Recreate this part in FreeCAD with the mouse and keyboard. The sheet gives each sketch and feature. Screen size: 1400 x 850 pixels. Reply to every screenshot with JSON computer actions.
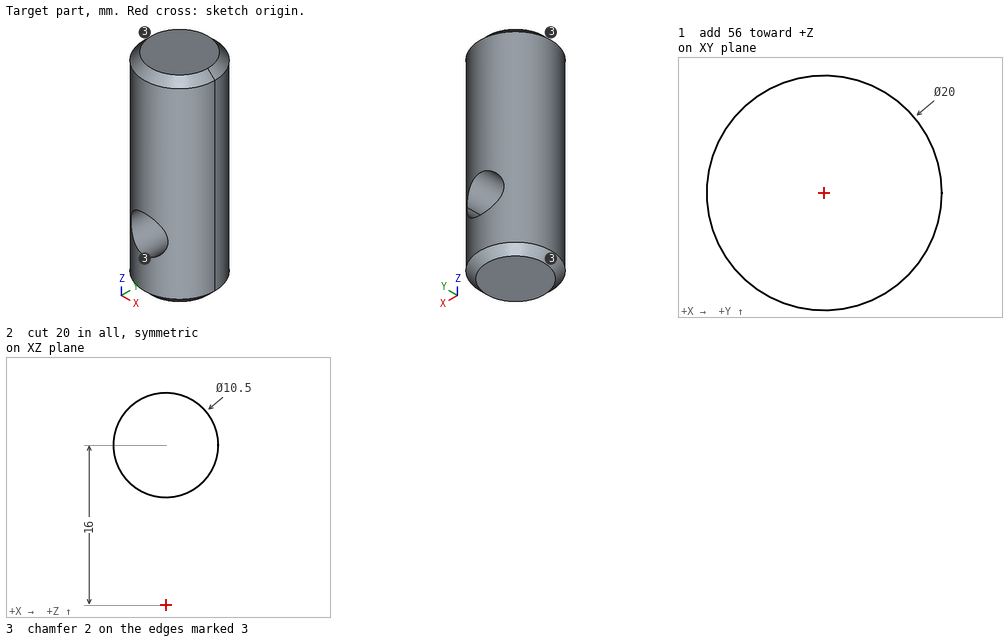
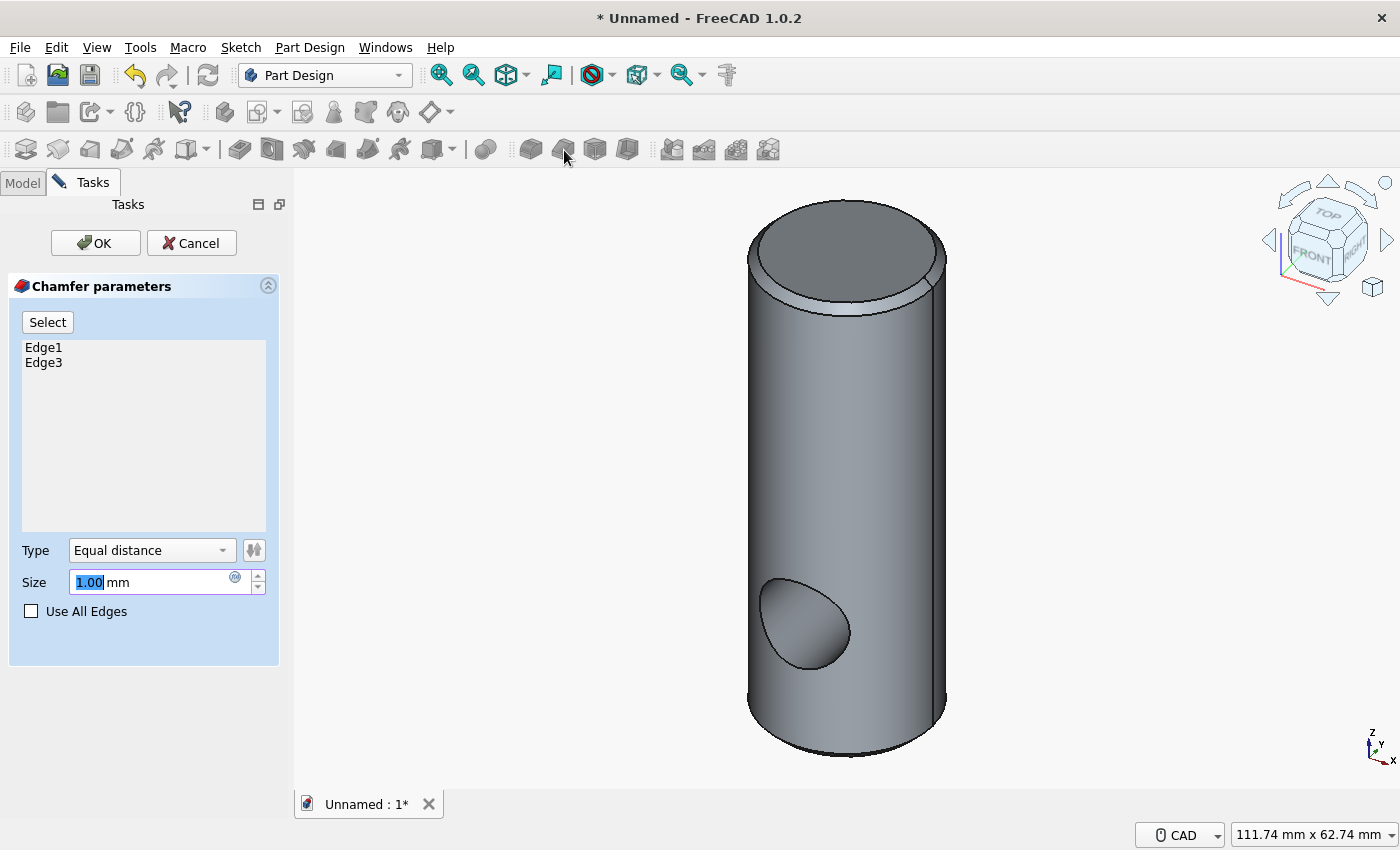
{"action": "type", "text": "2"}
{"action": "key", "text": "Tab"}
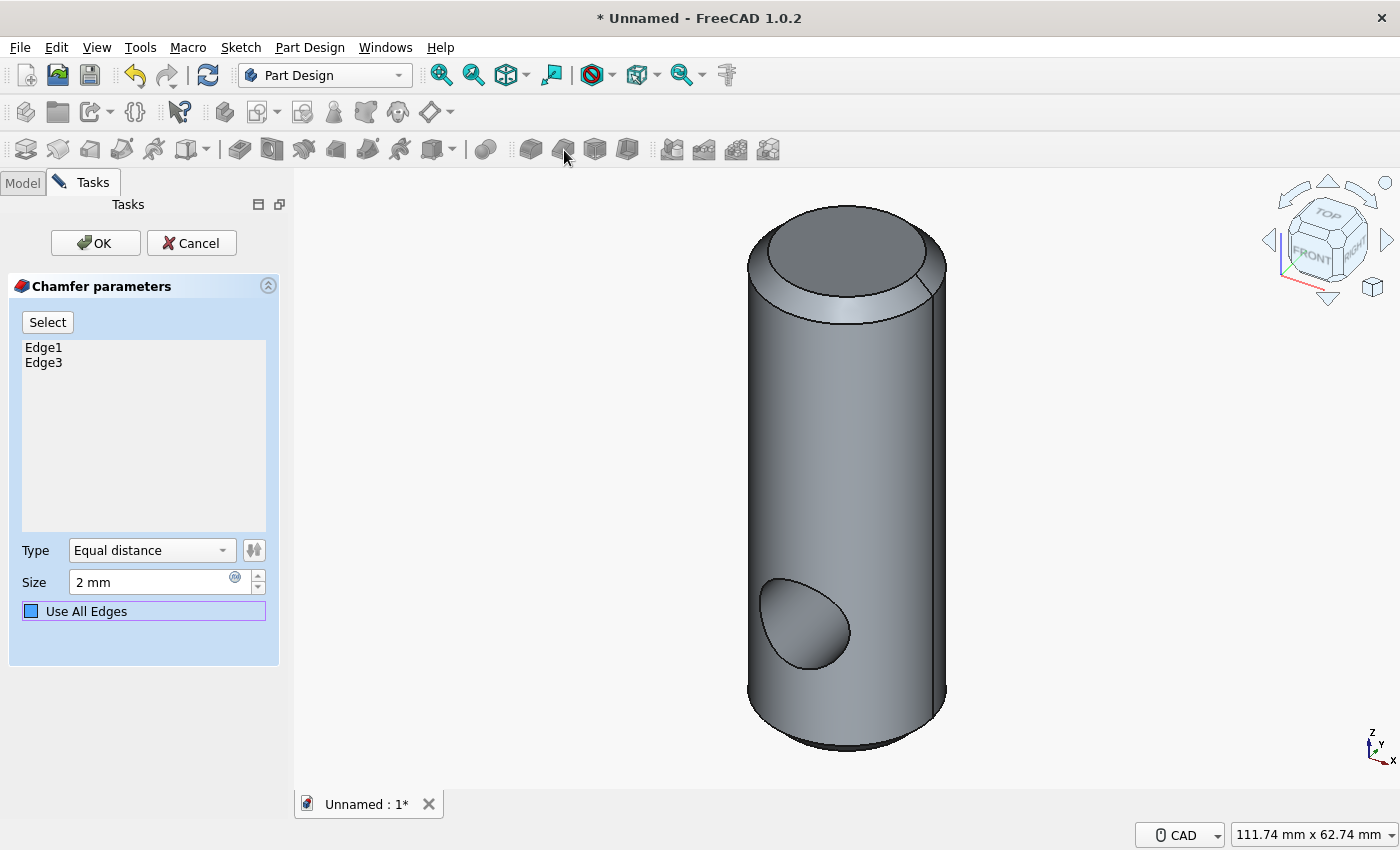
{"action": "left_click", "coordinate": [96, 243]}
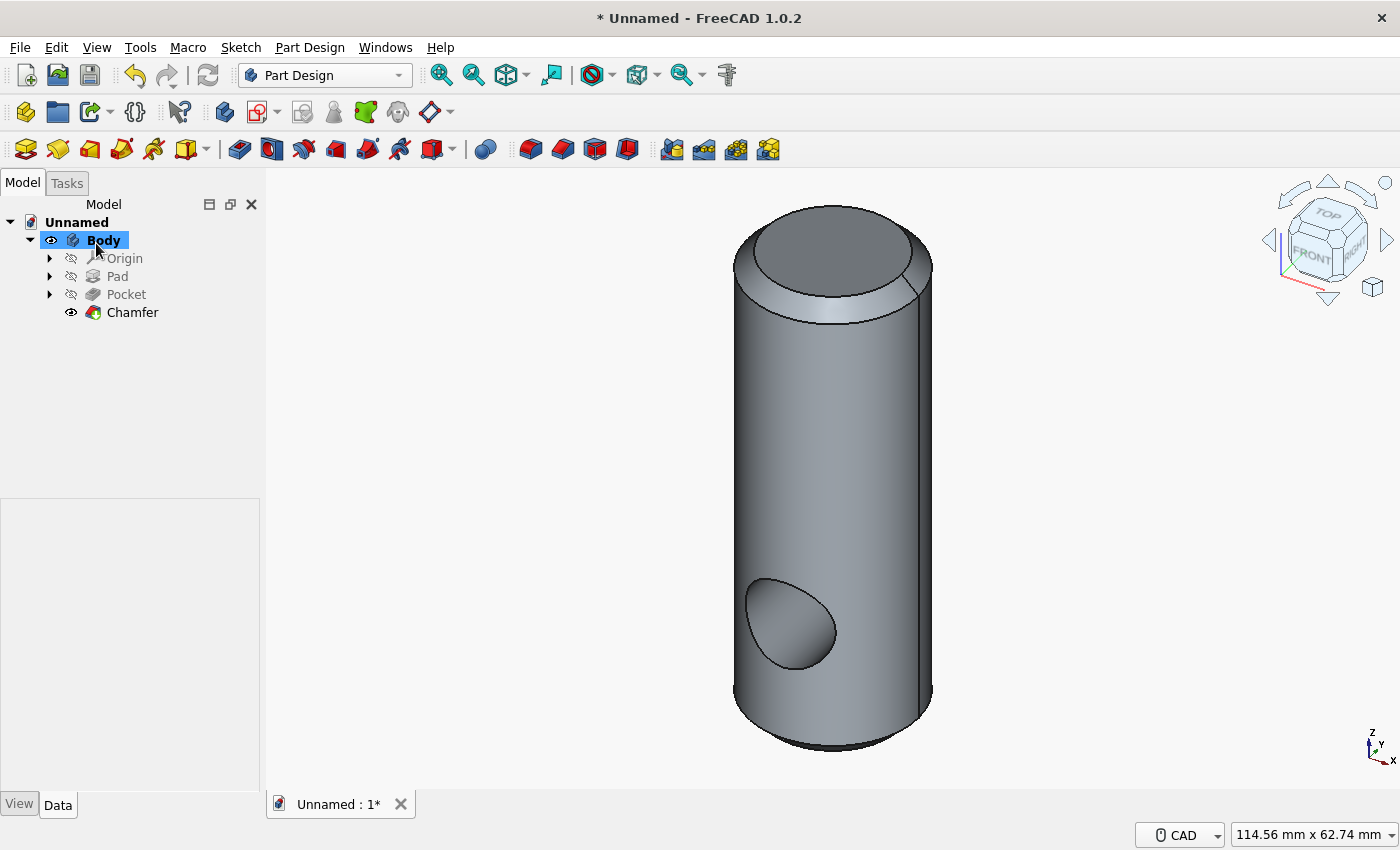
{"action": "key", "text": "0"}